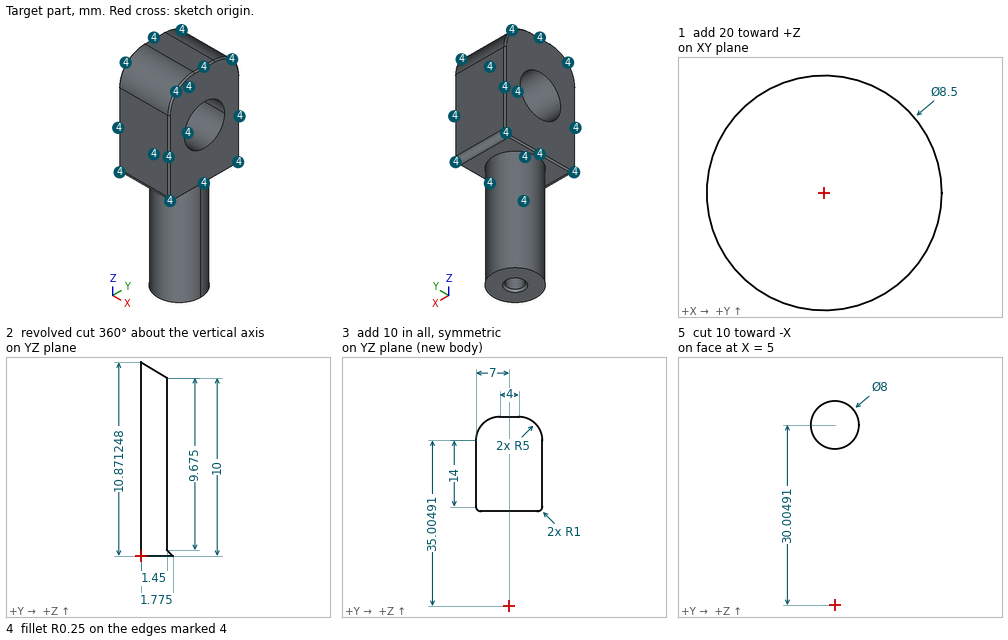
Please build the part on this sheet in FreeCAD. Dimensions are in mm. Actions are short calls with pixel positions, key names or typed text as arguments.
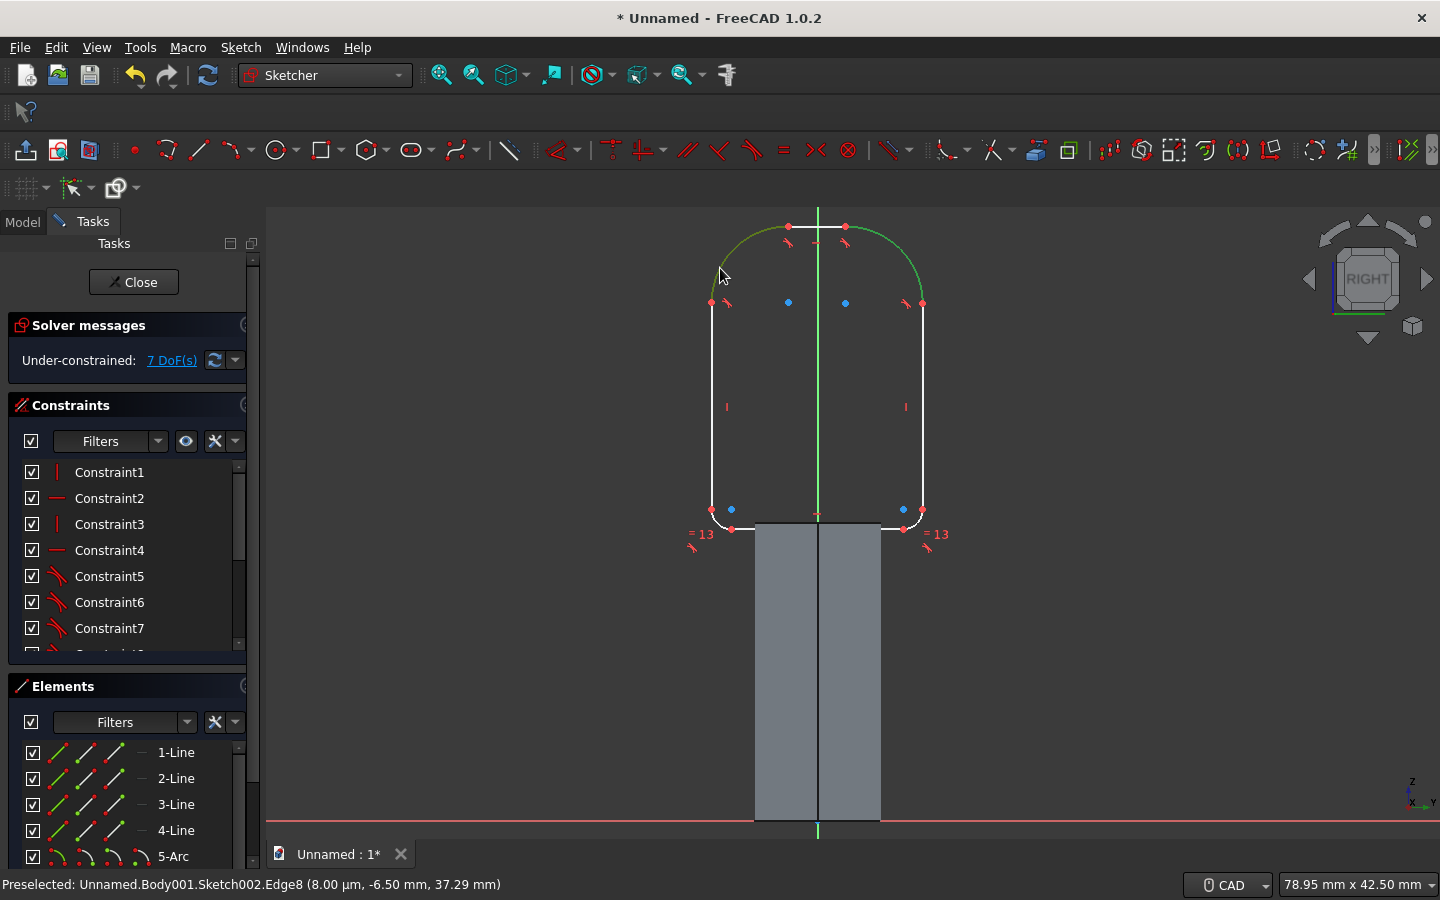
click(784, 150)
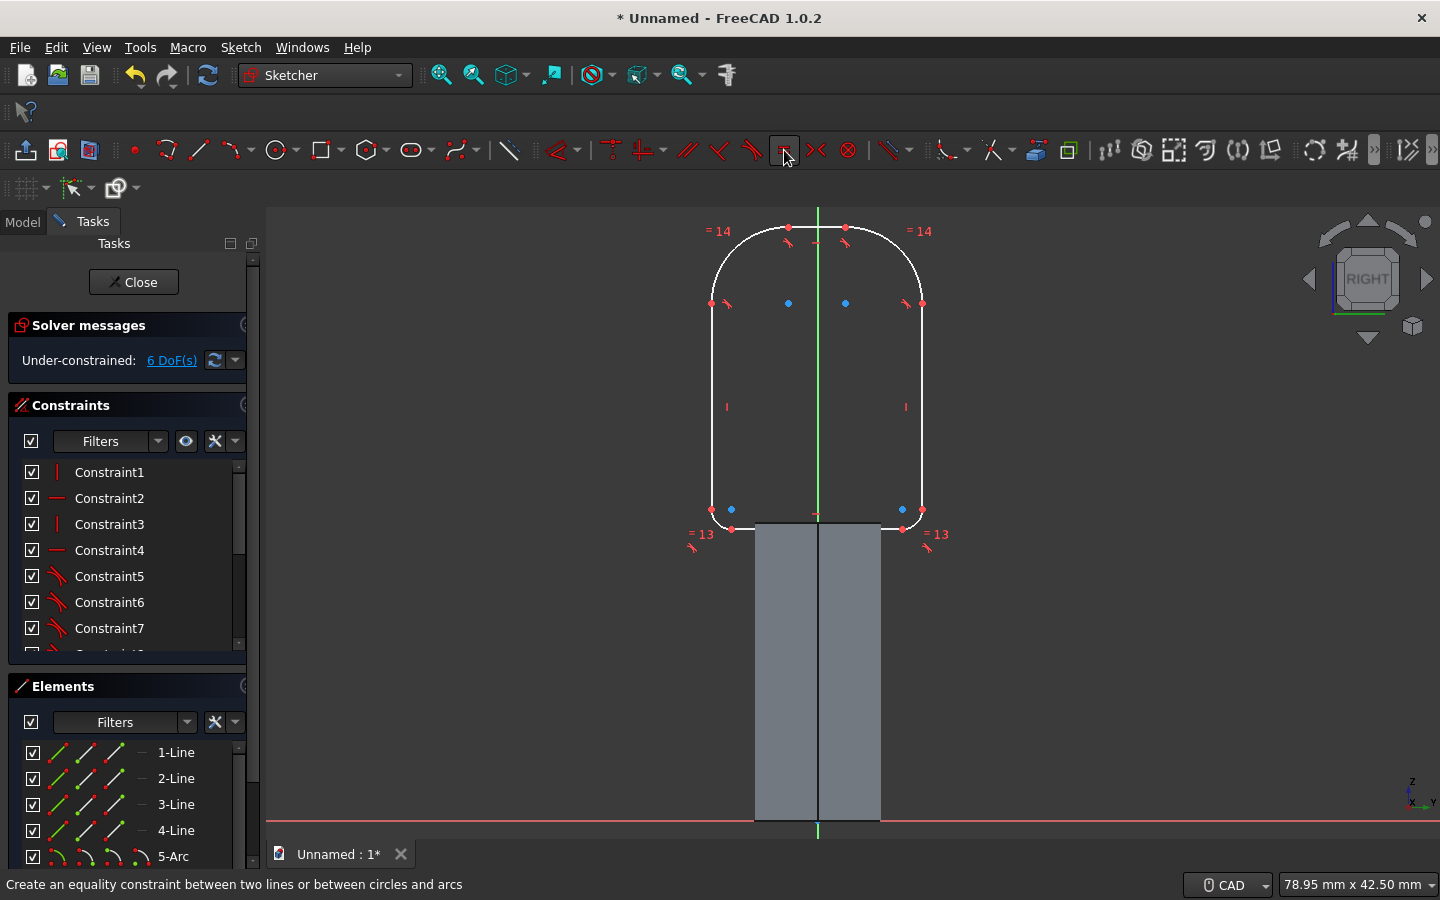
click(556, 150)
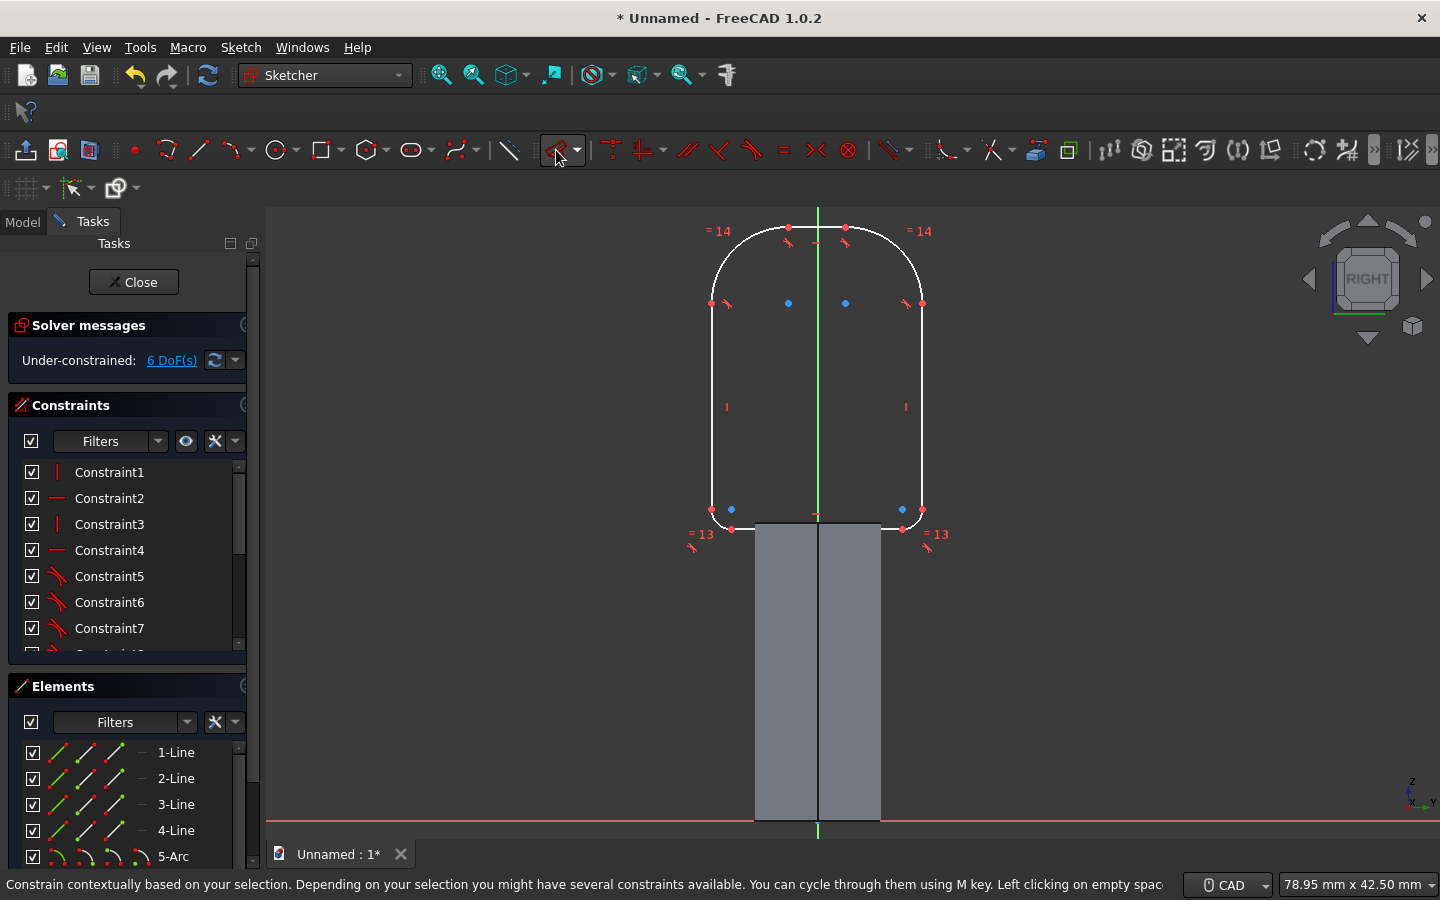
scroll(714, 519, up, 5)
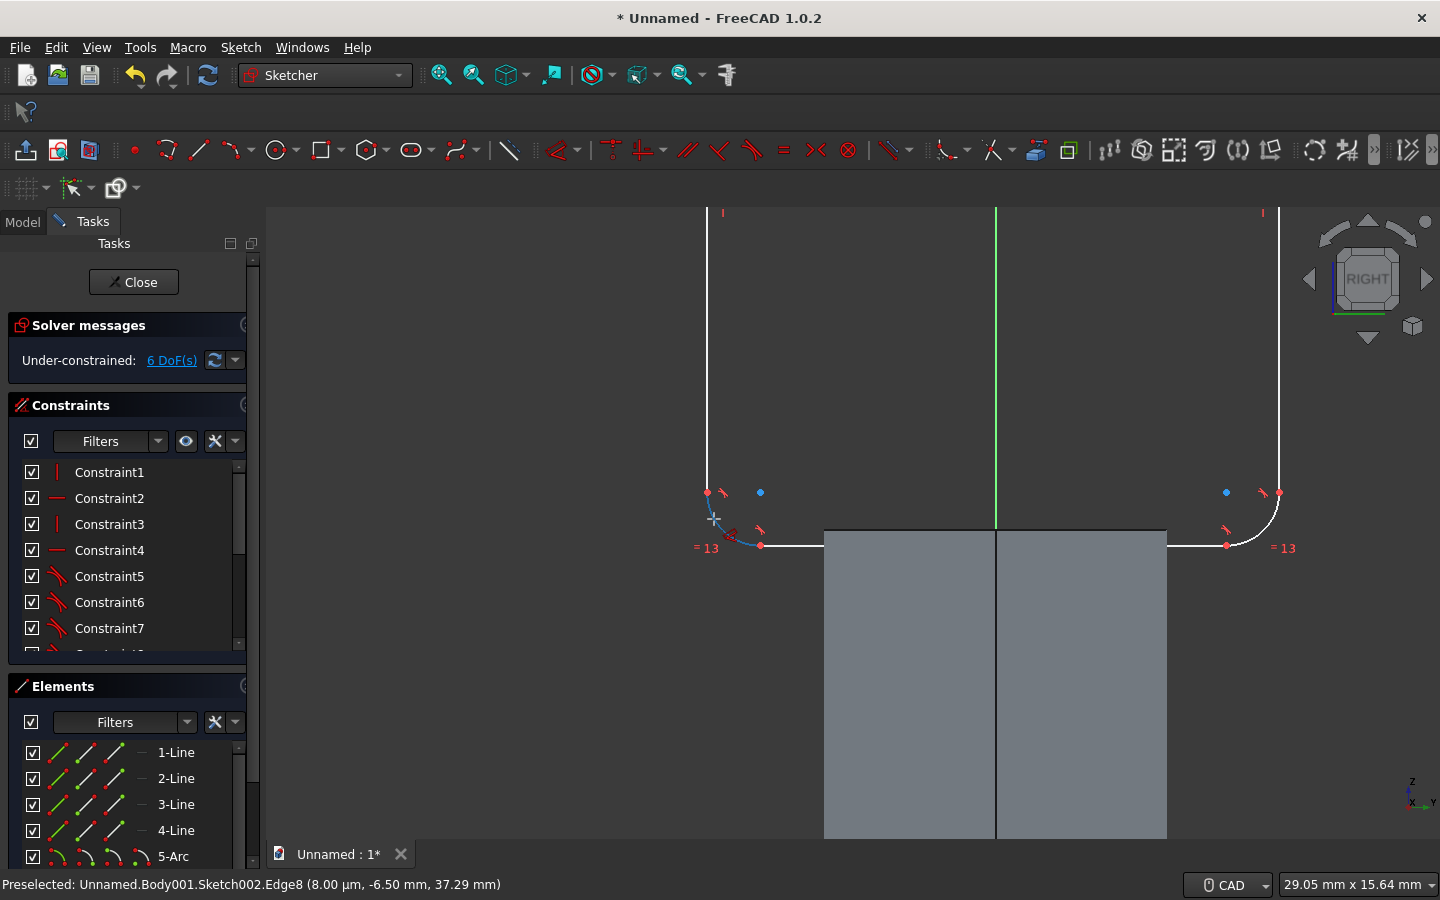
click(713, 517)
click(685, 532)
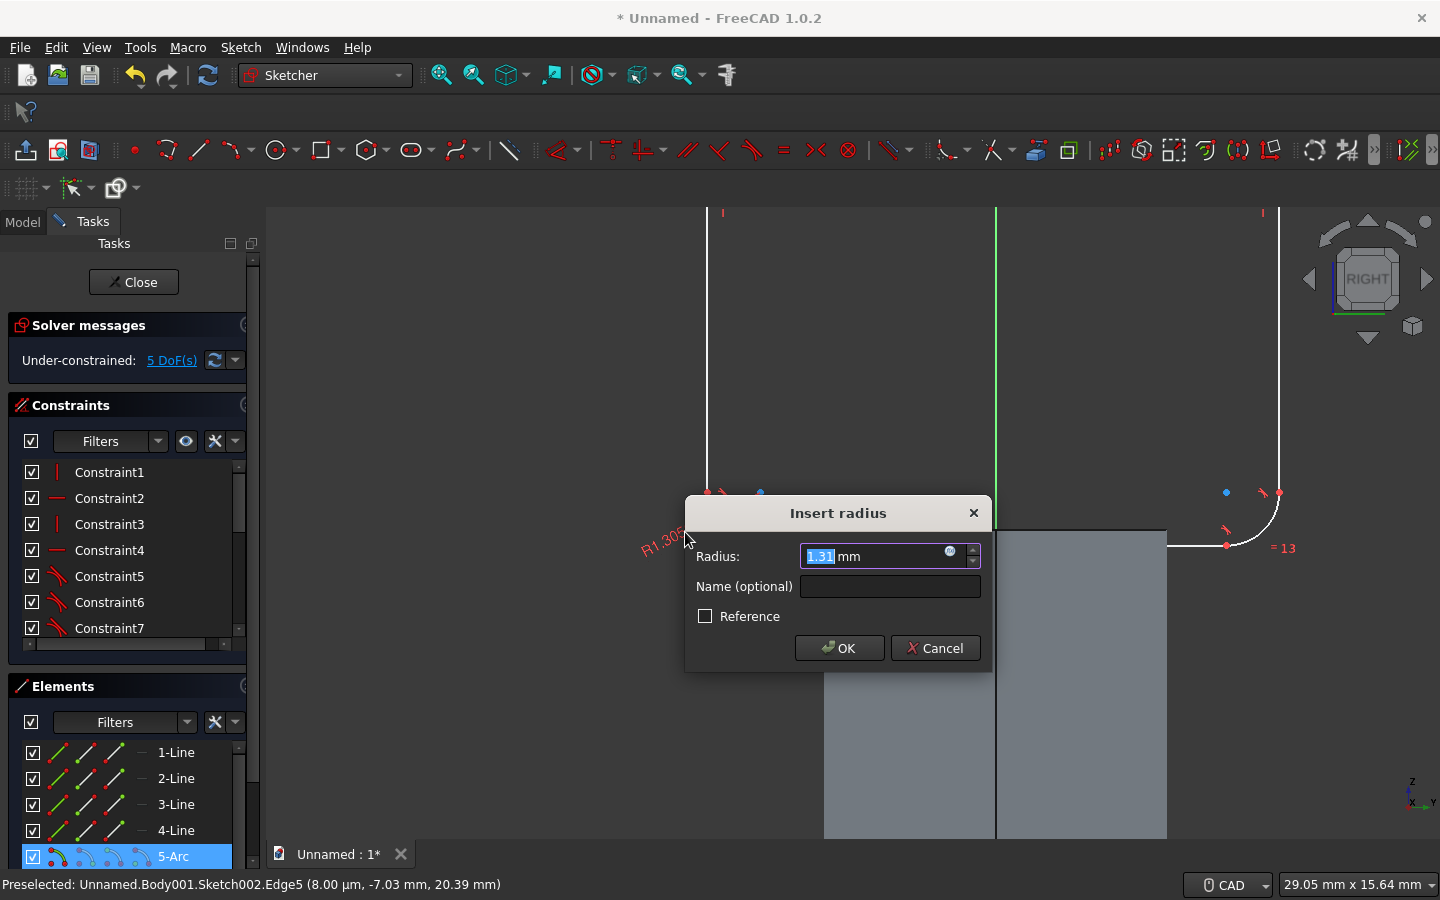
text(1)
key(Return)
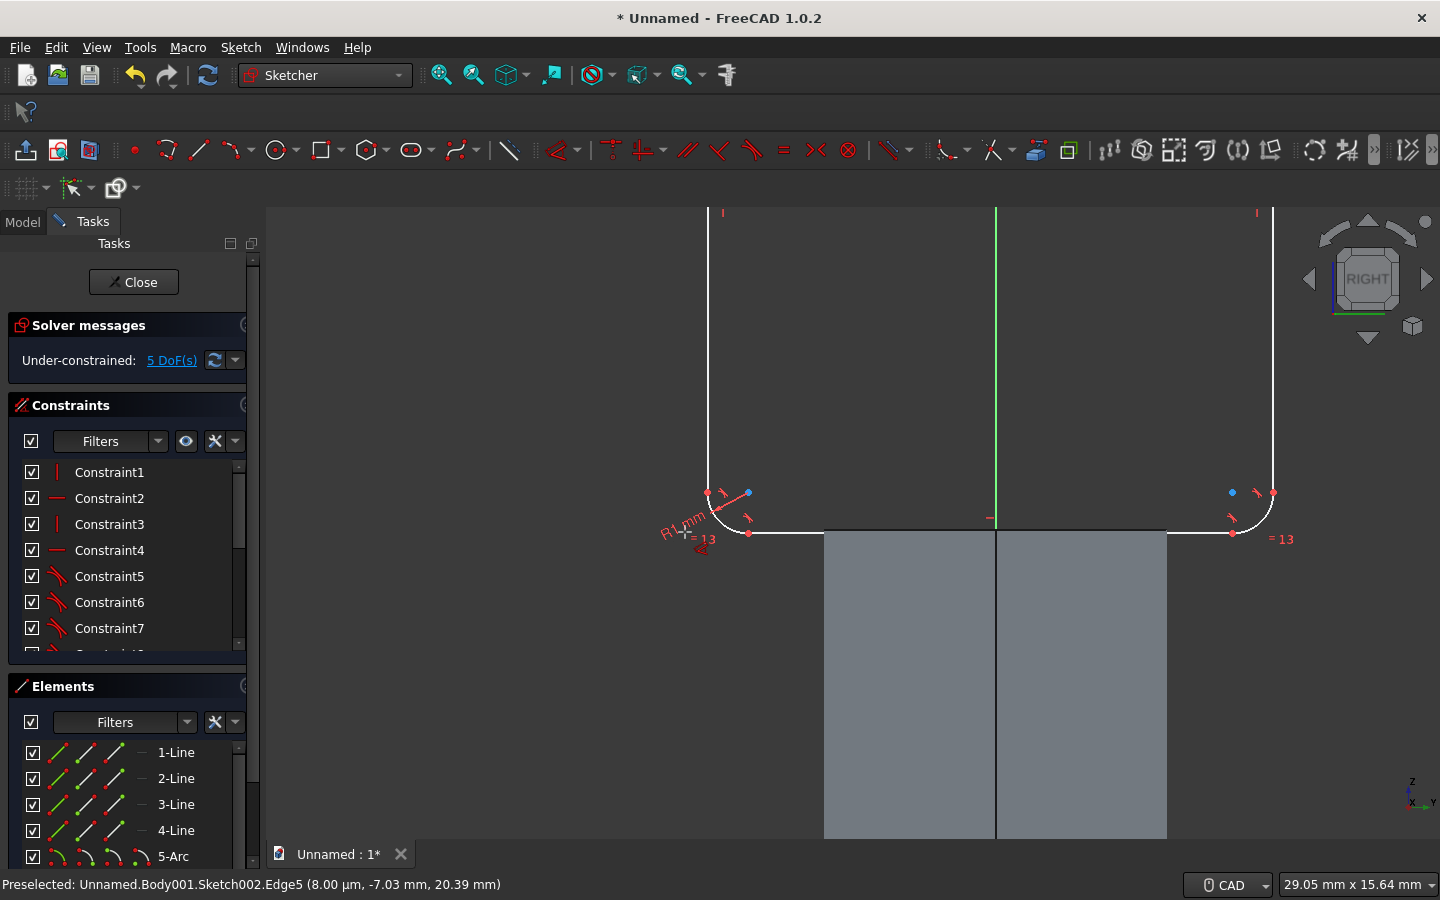
scroll(715, 521, down, 7)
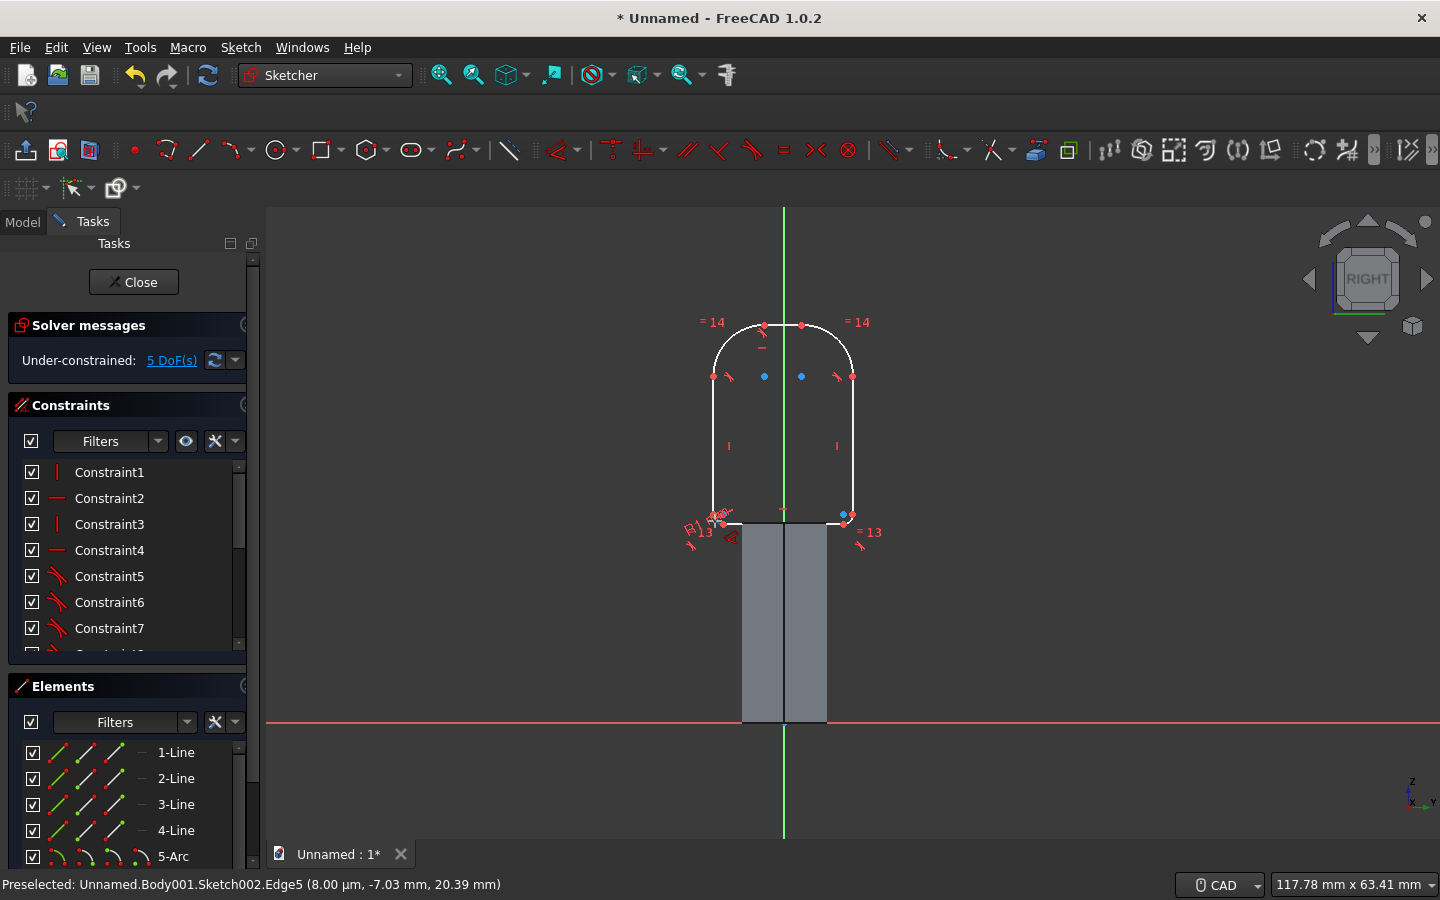
click(847, 353)
click(875, 338)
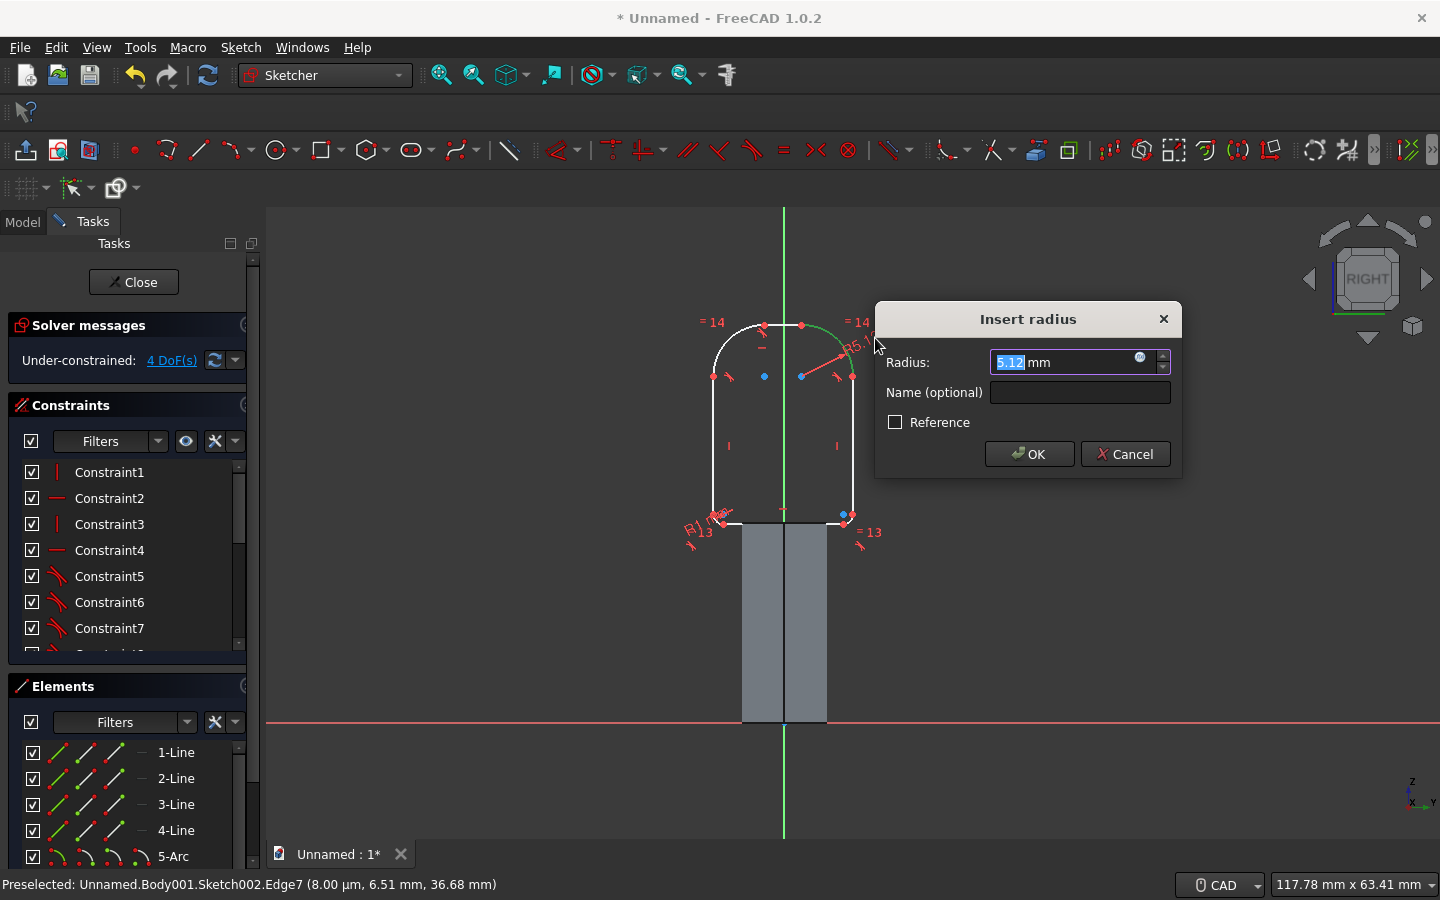
text(5)
key(Return)